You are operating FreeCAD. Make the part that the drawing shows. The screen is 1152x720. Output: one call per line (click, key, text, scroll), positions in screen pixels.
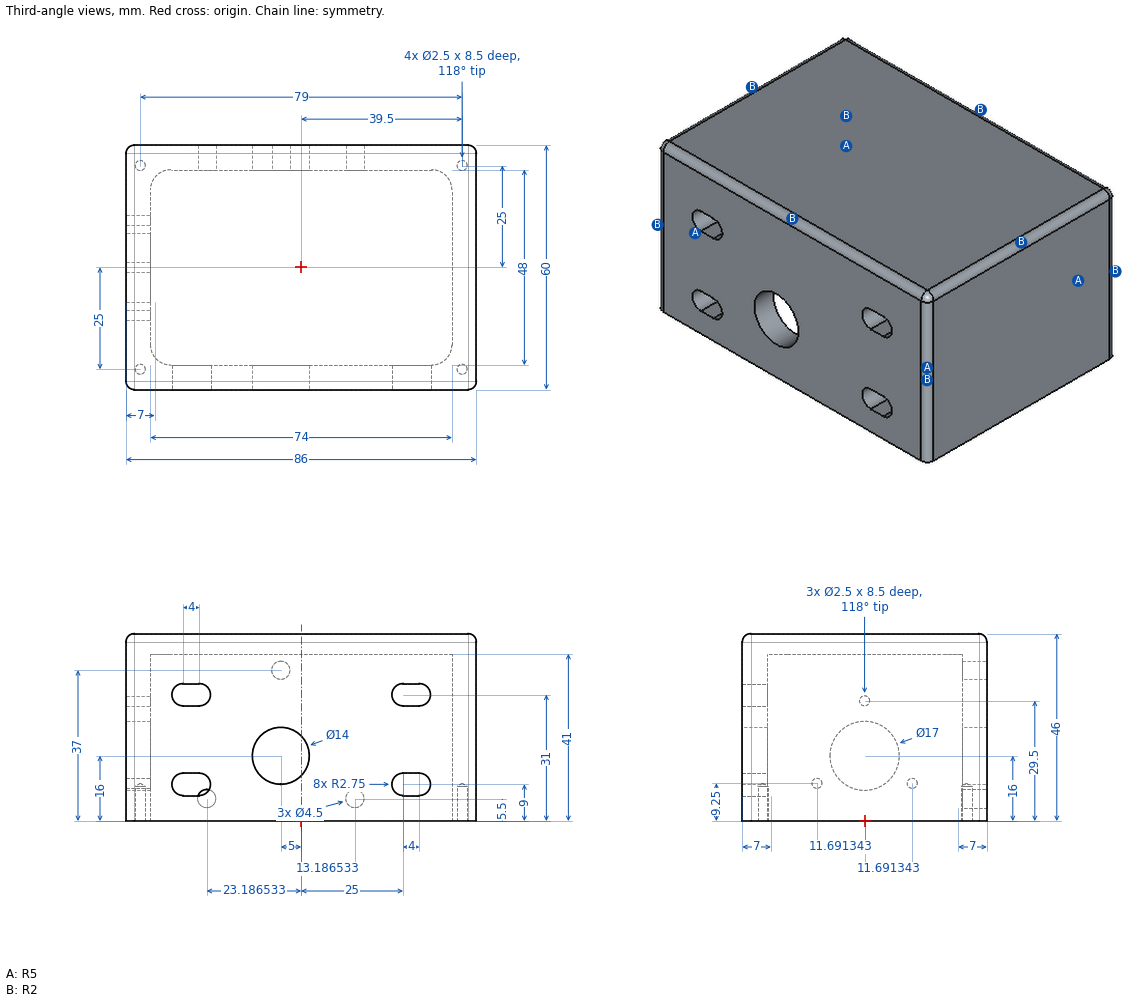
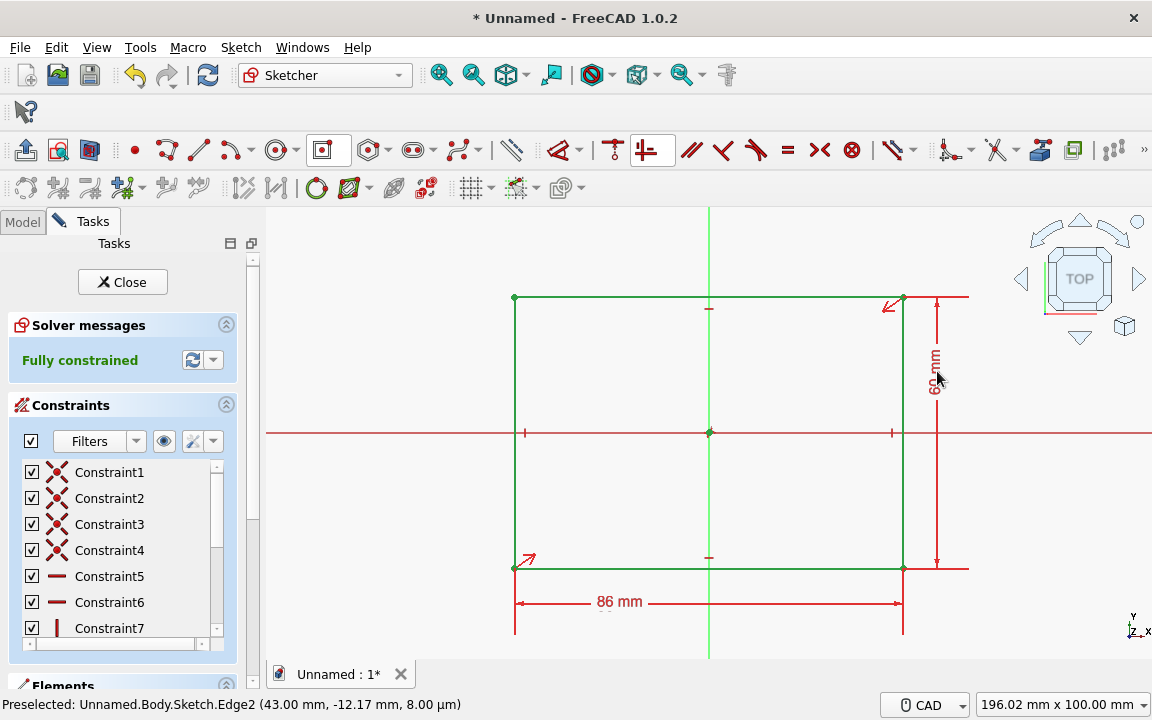
click(123, 282)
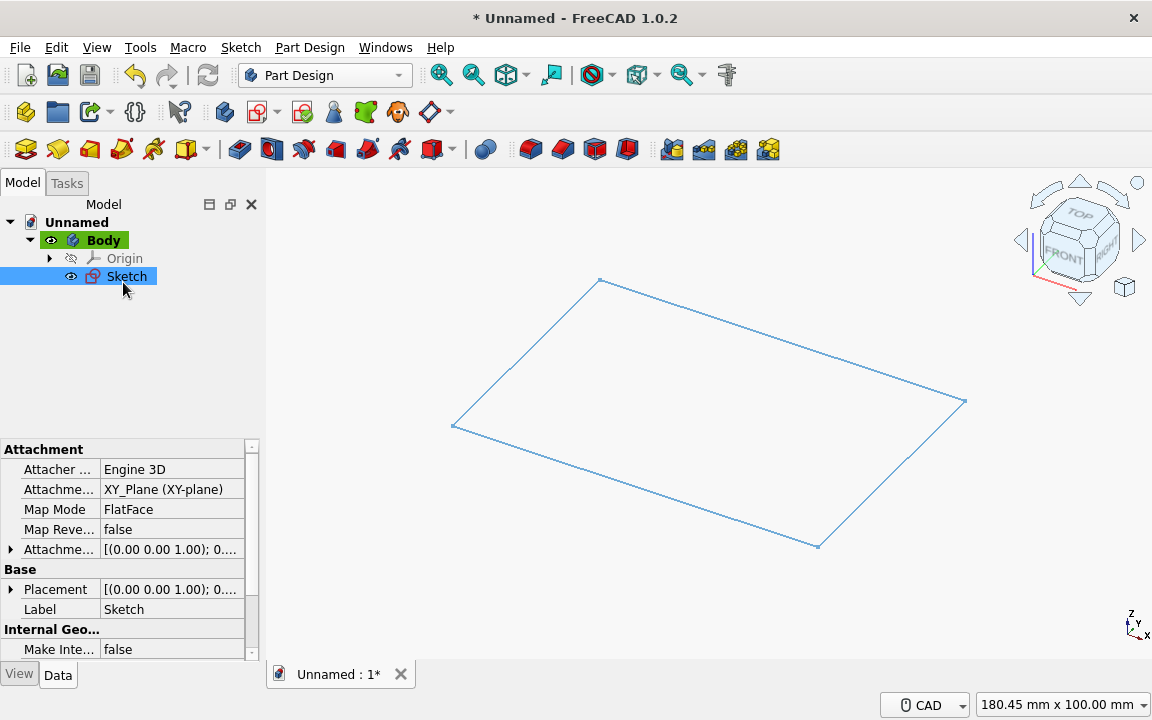
click(26, 150)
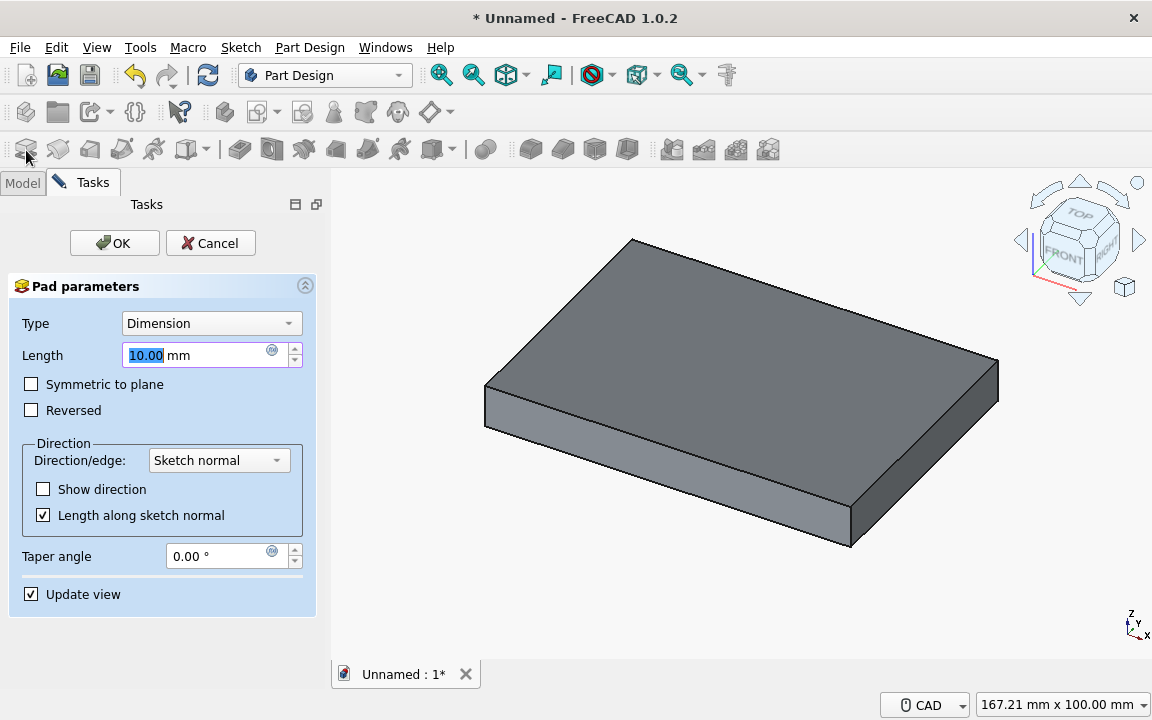
text(46)
key(Tab)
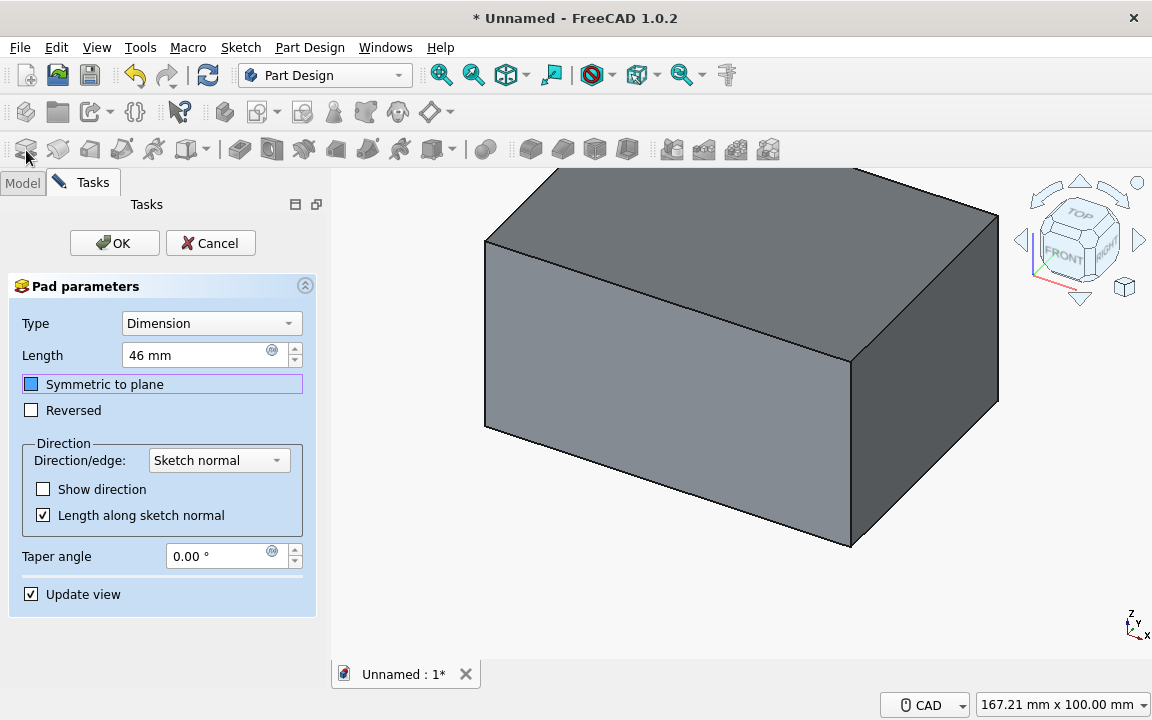
click(115, 243)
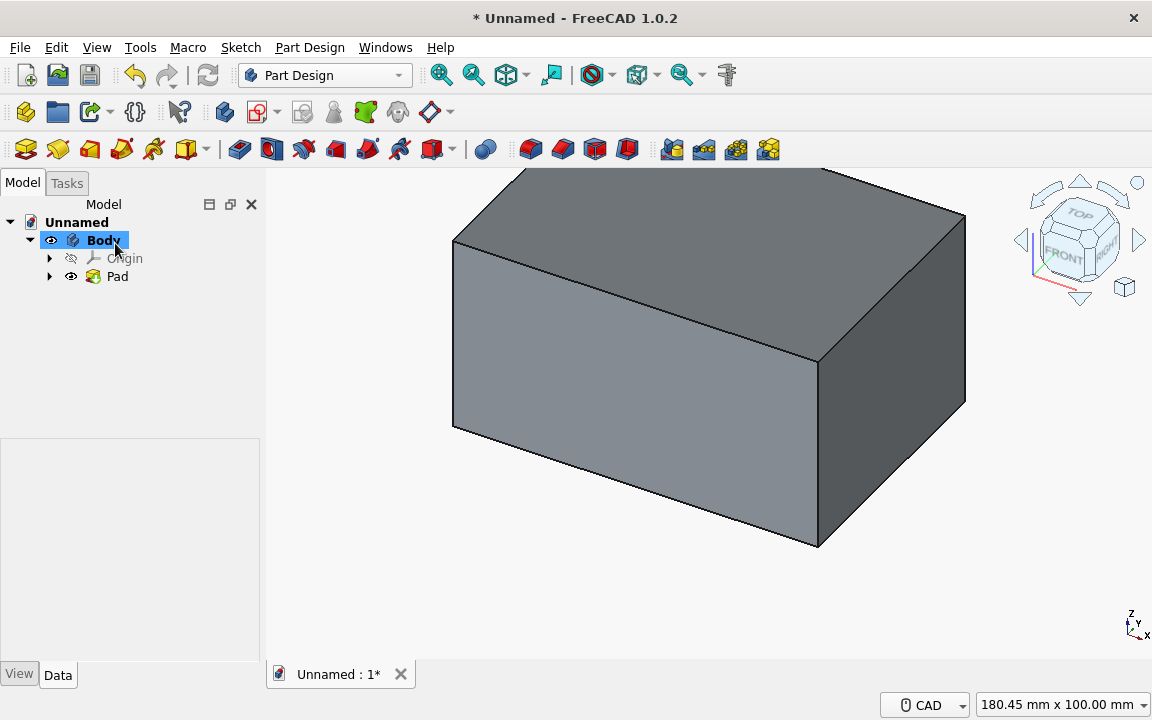
key(v)
key(f)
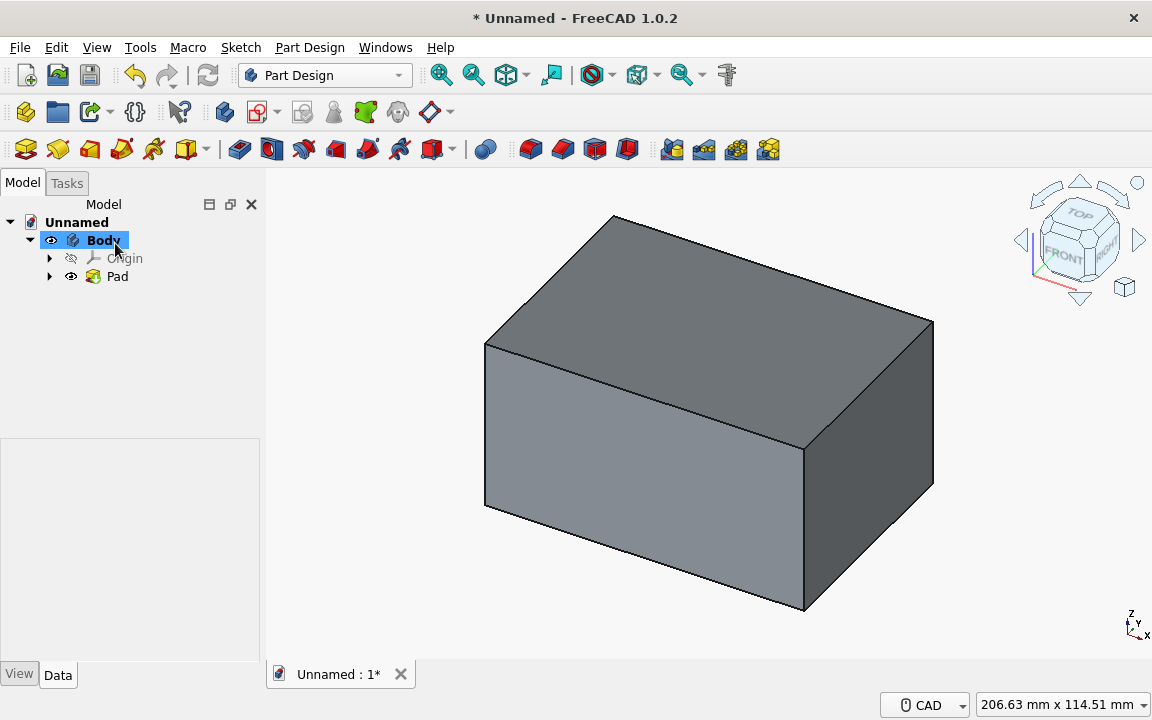
click(258, 112)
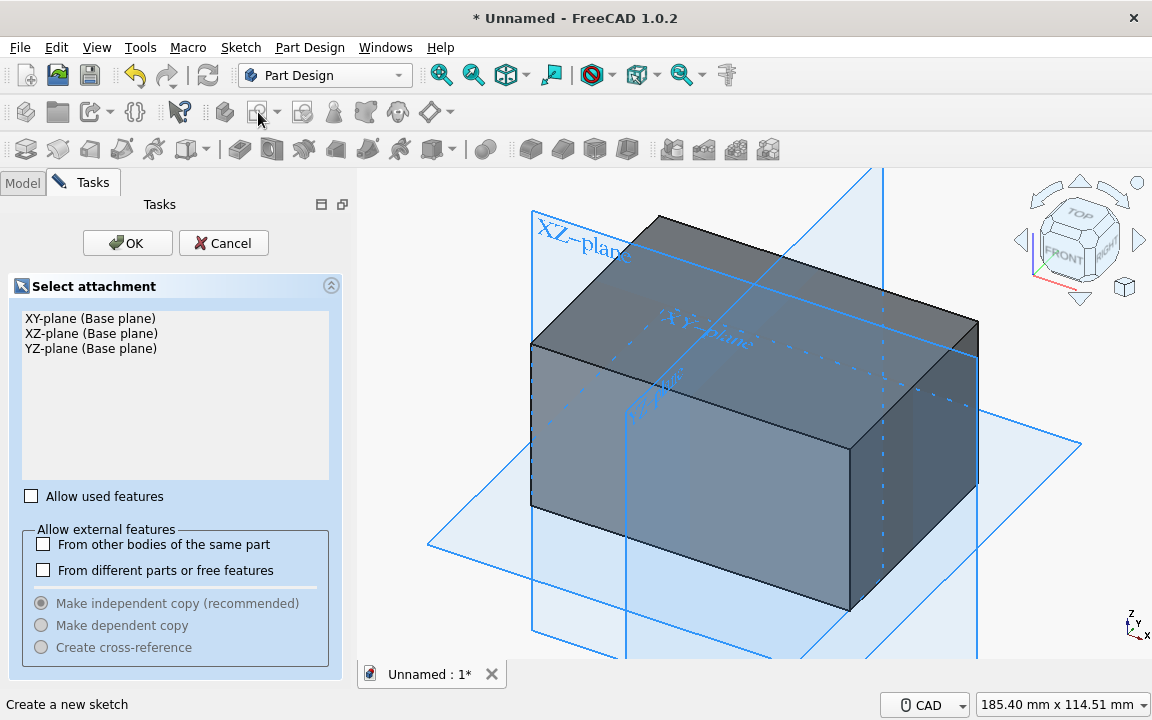
click(82, 318)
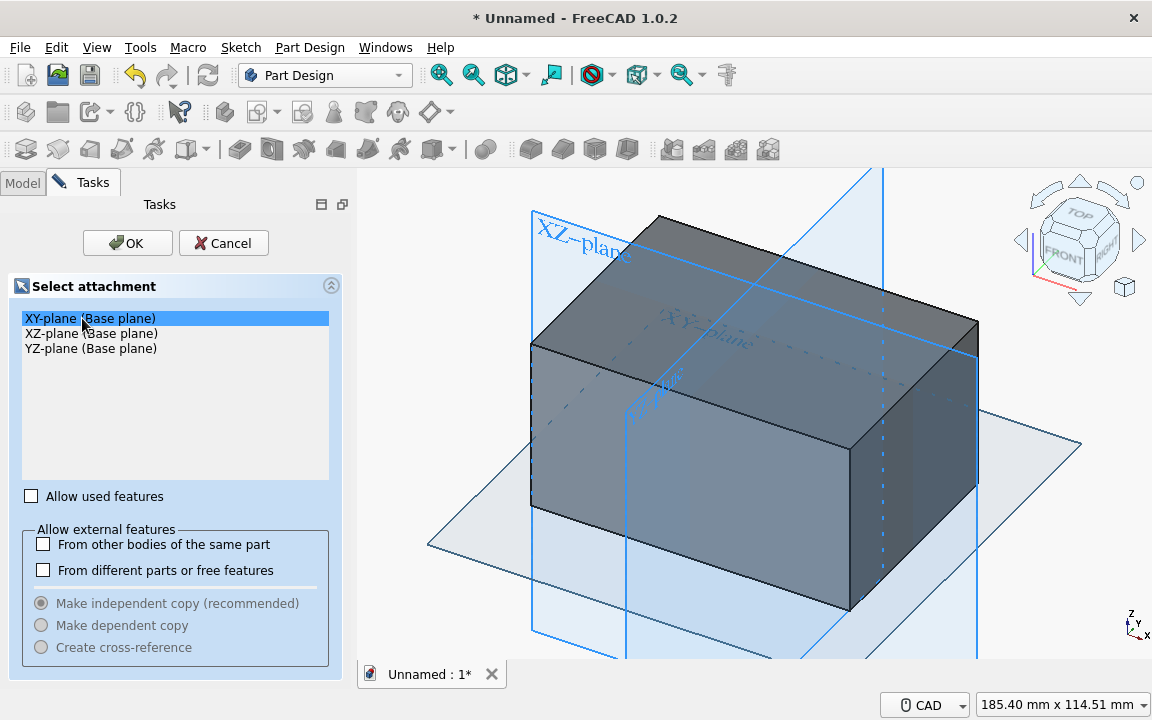
click(128, 243)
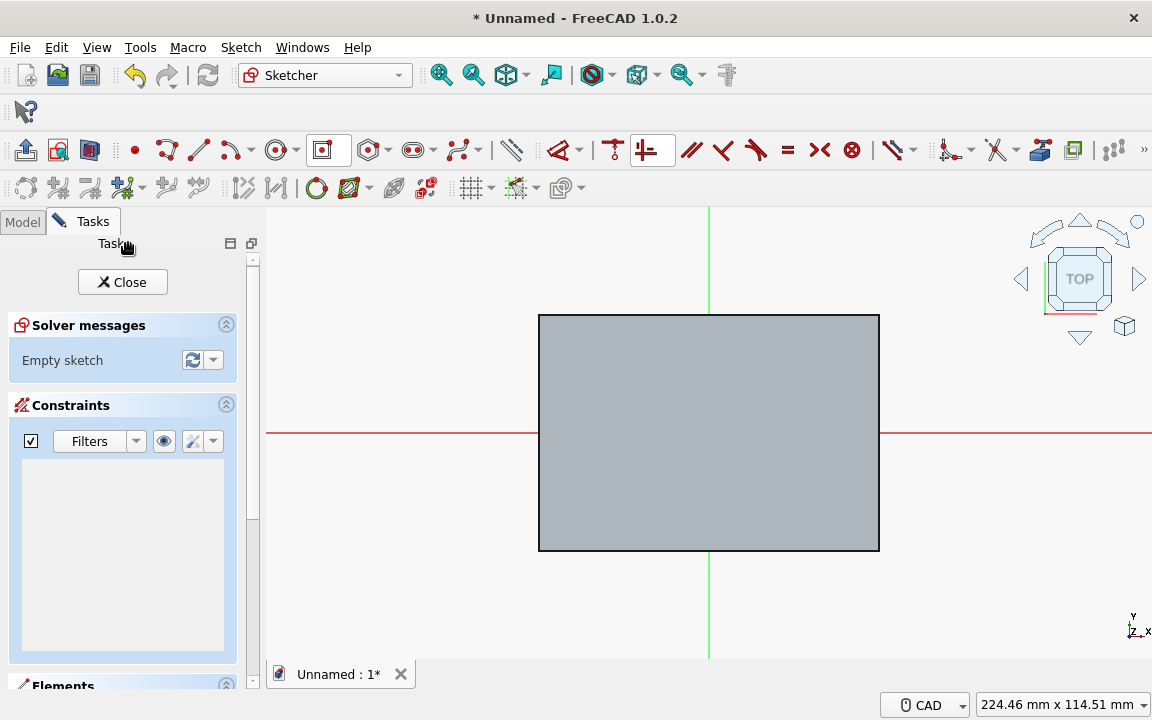
click(90, 150)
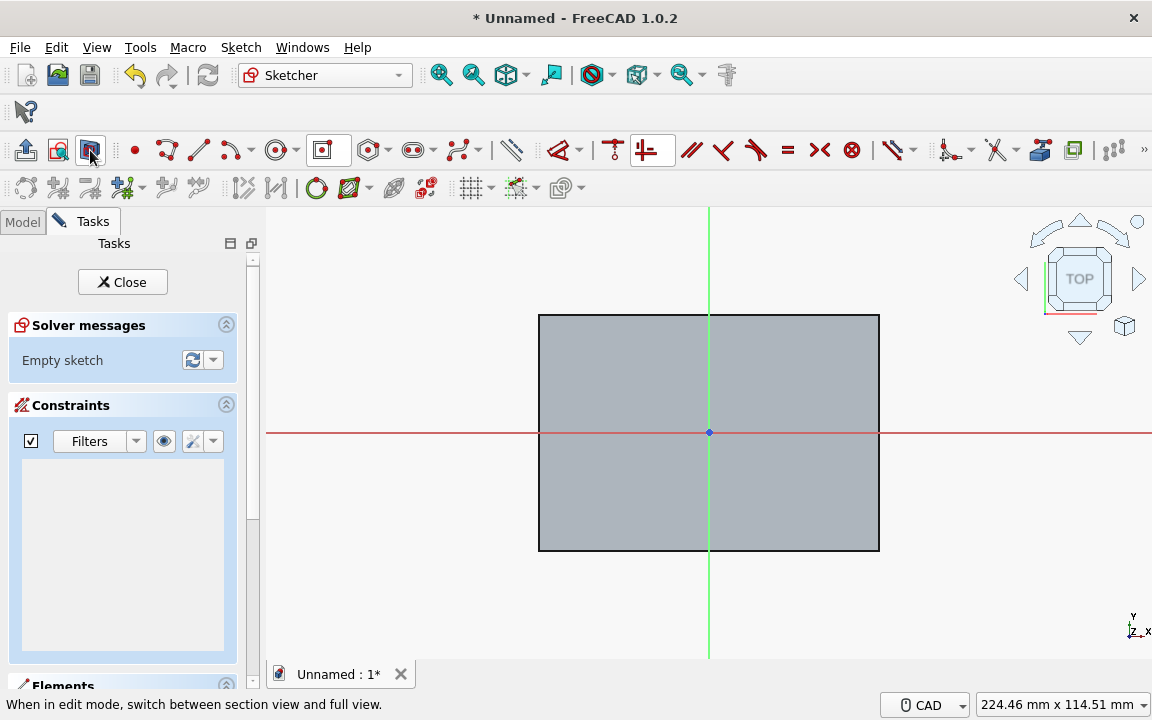
scroll(848, 433, up, 2)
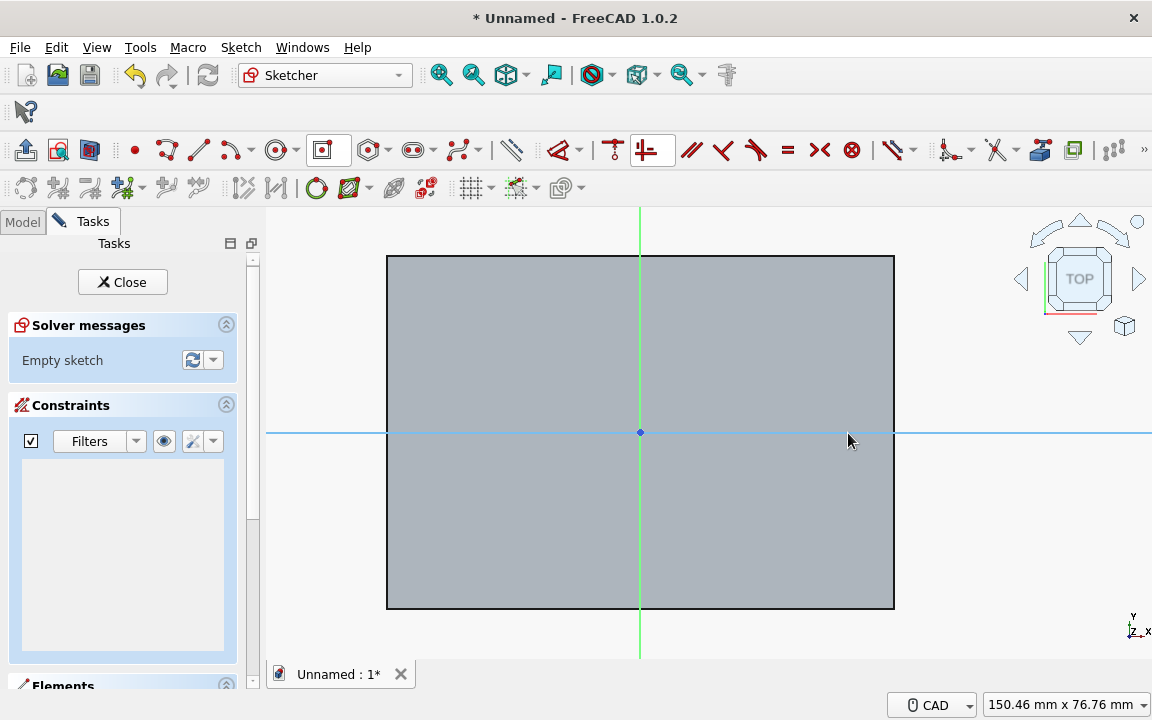
key(g)
key(v)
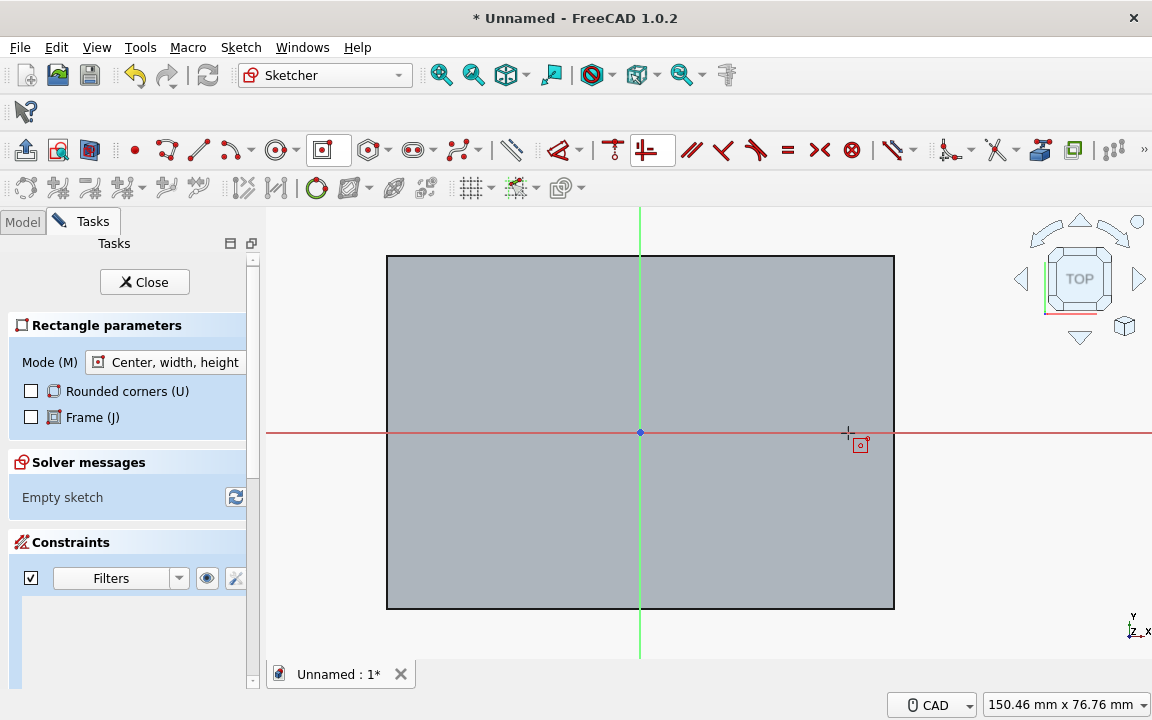
click(640, 433)
click(858, 291)
key(Escape)